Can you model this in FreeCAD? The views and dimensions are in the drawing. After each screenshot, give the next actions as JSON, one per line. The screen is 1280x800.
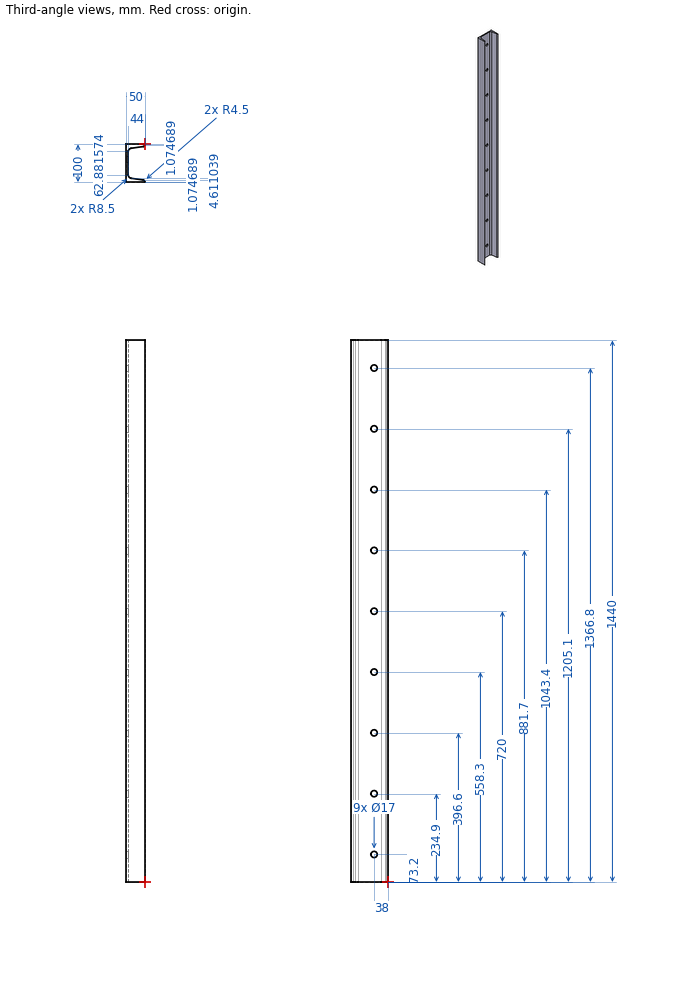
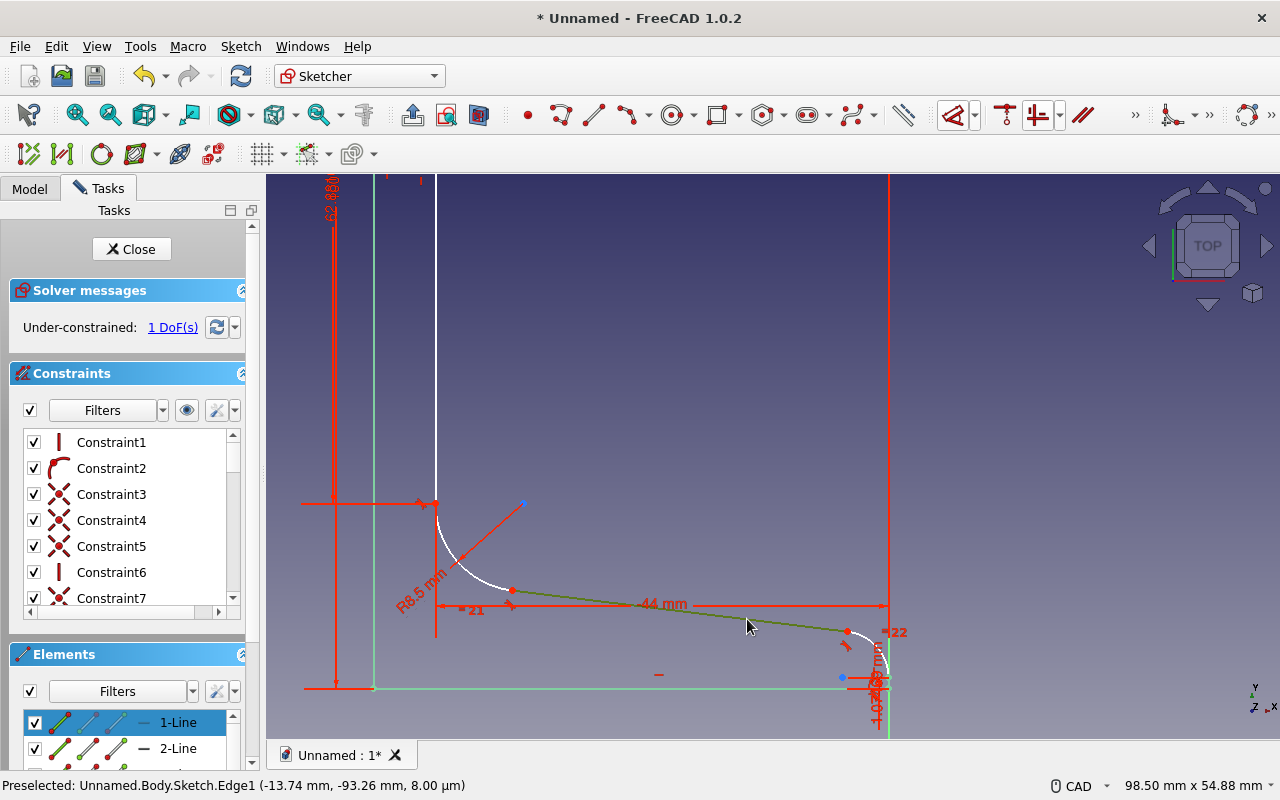
{"action": "left_click", "coordinate": [974, 116]}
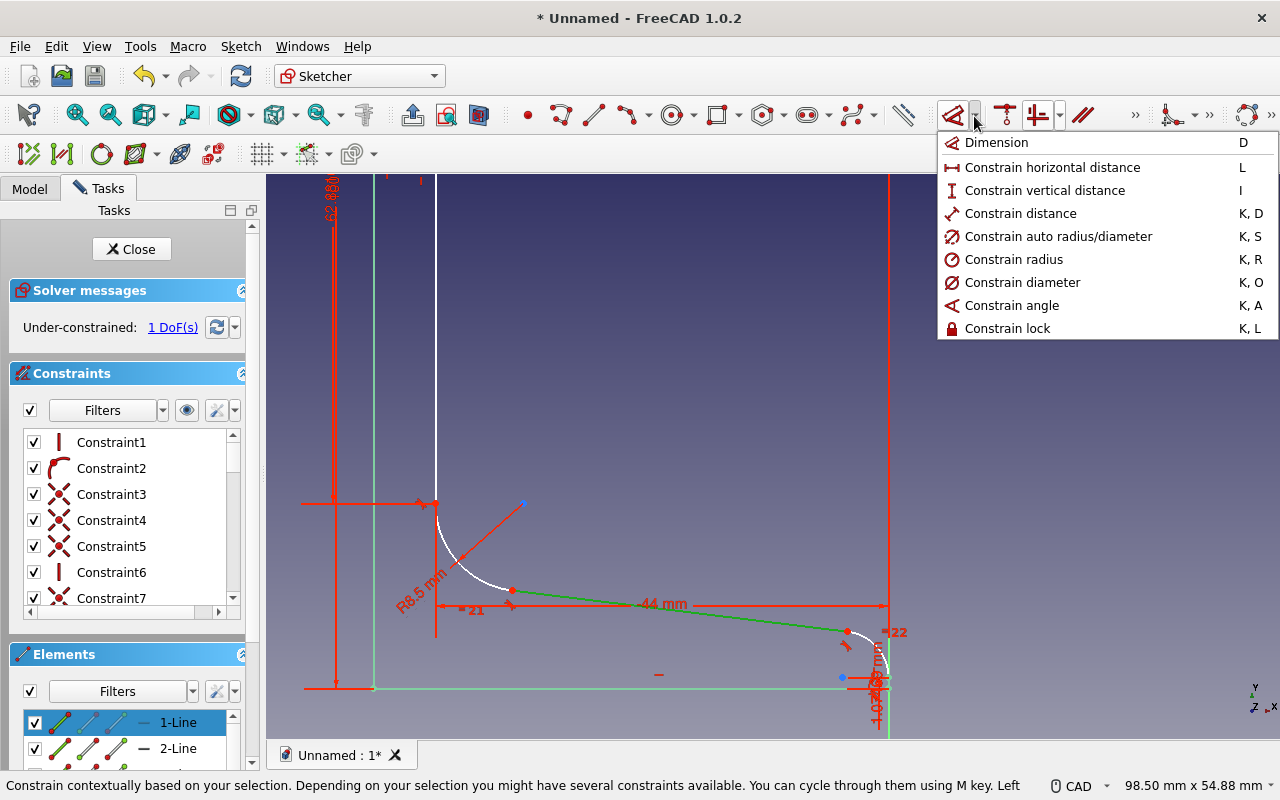
{"action": "left_click", "coordinate": [1108, 190]}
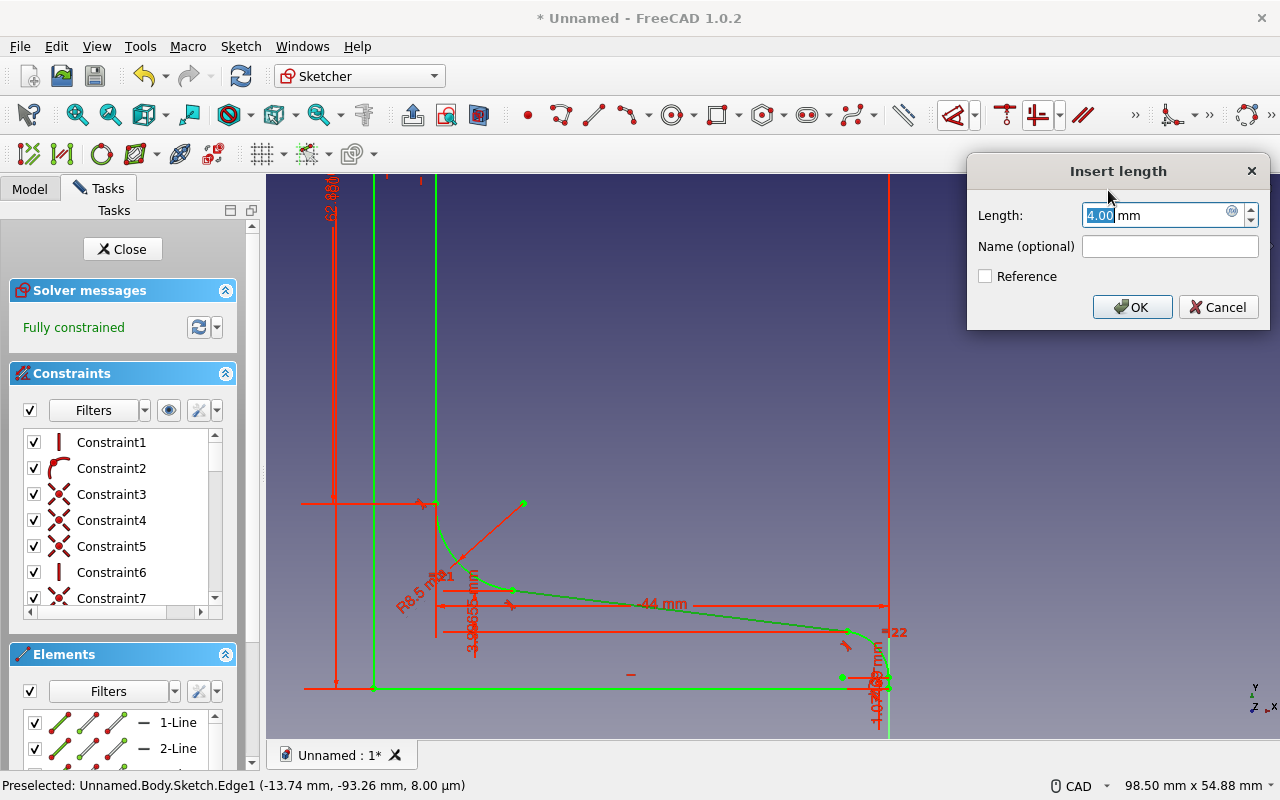
{"action": "type", "text": "4.611039"}
{"action": "key", "text": "Return"}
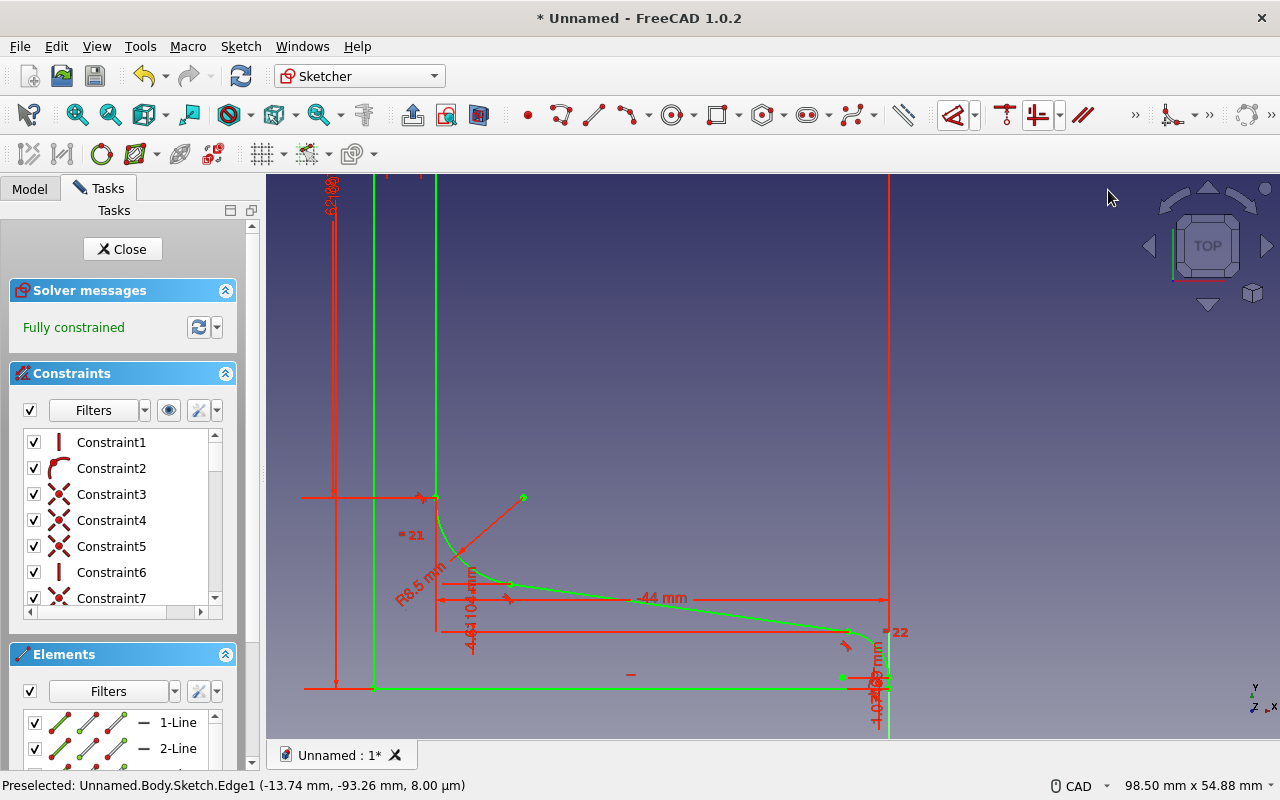
{"action": "left_click", "coordinate": [123, 249]}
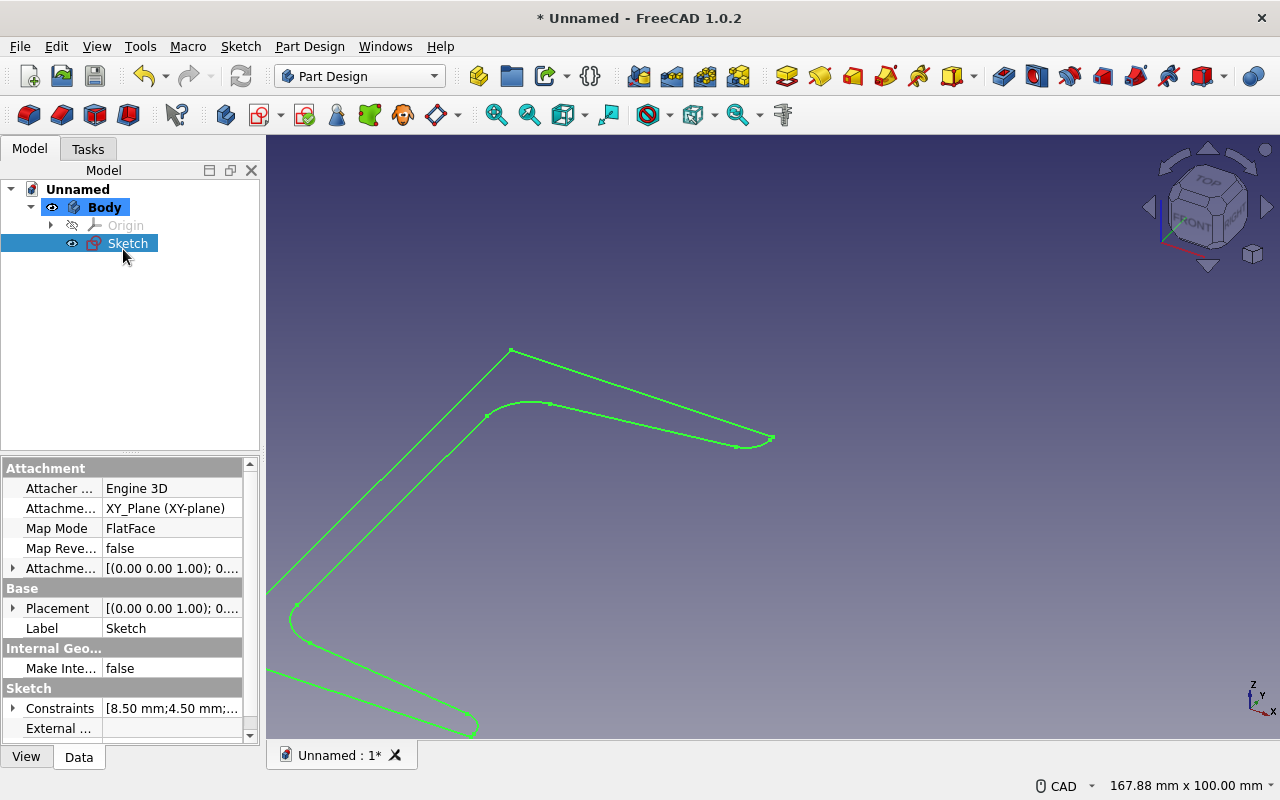
{"action": "left_click", "coordinate": [787, 76]}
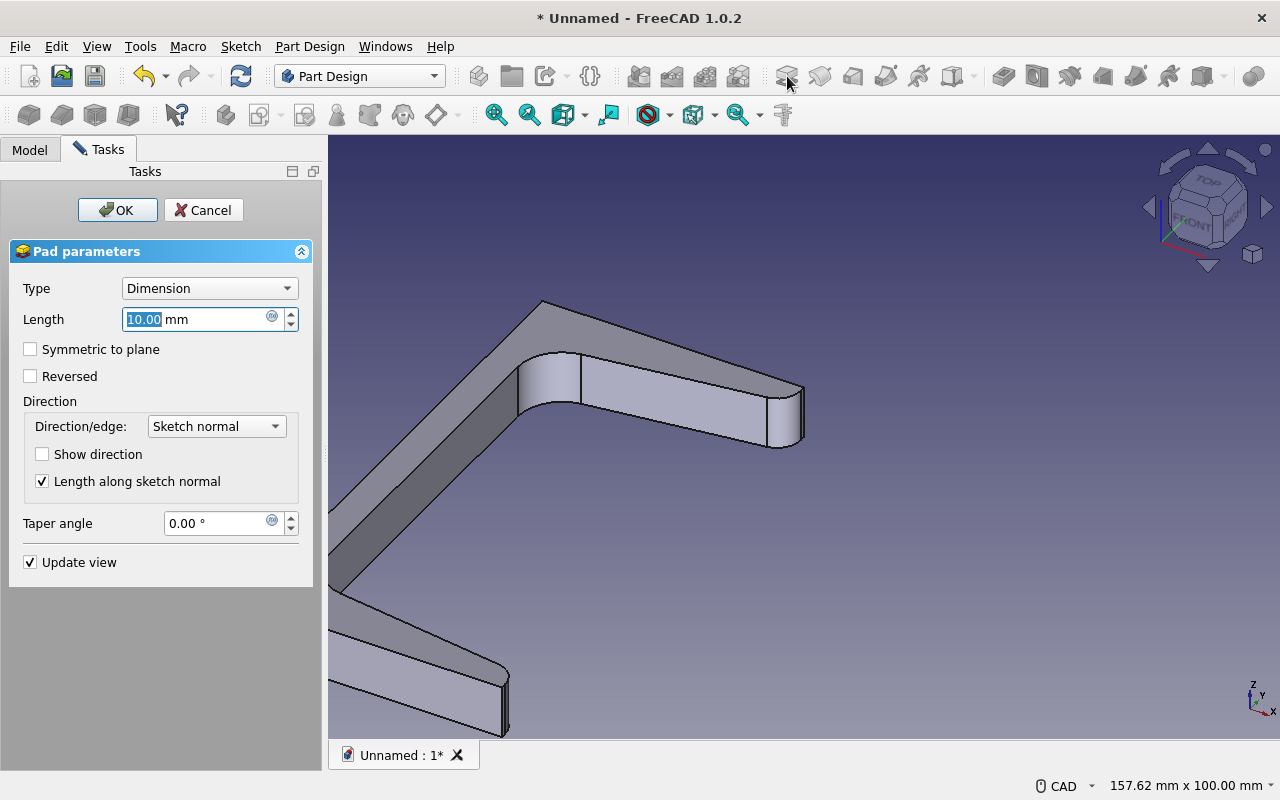
{"action": "type", "text": "1440"}
{"action": "key", "text": "Tab"}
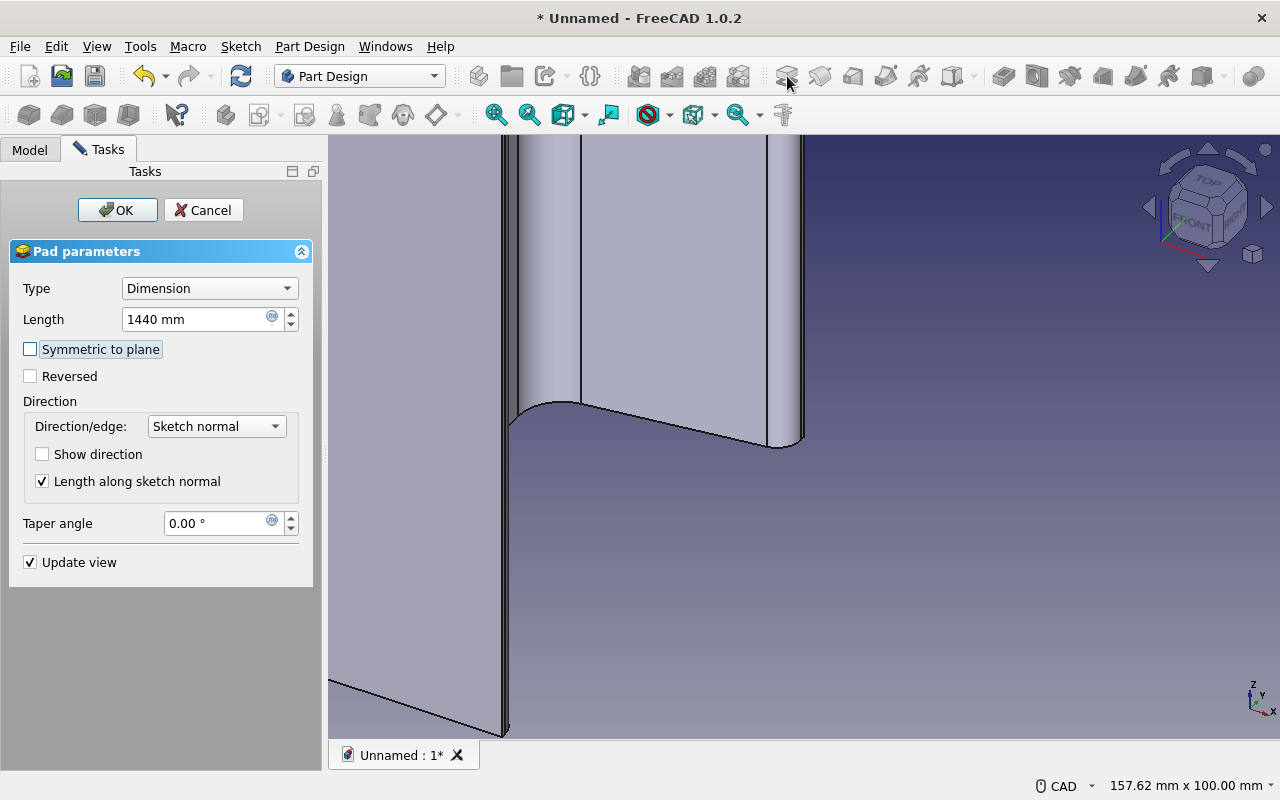
{"action": "left_click", "coordinate": [118, 210]}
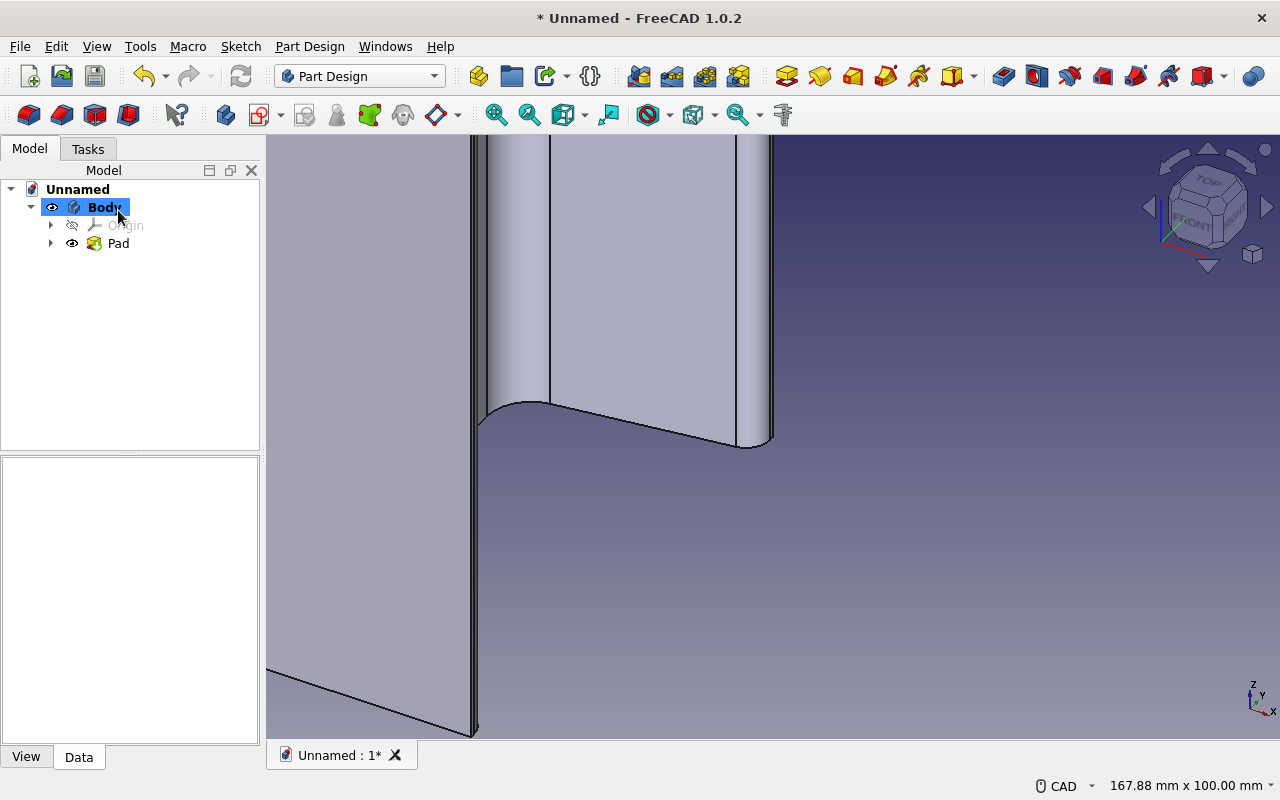
{"action": "left_click", "coordinate": [497, 116]}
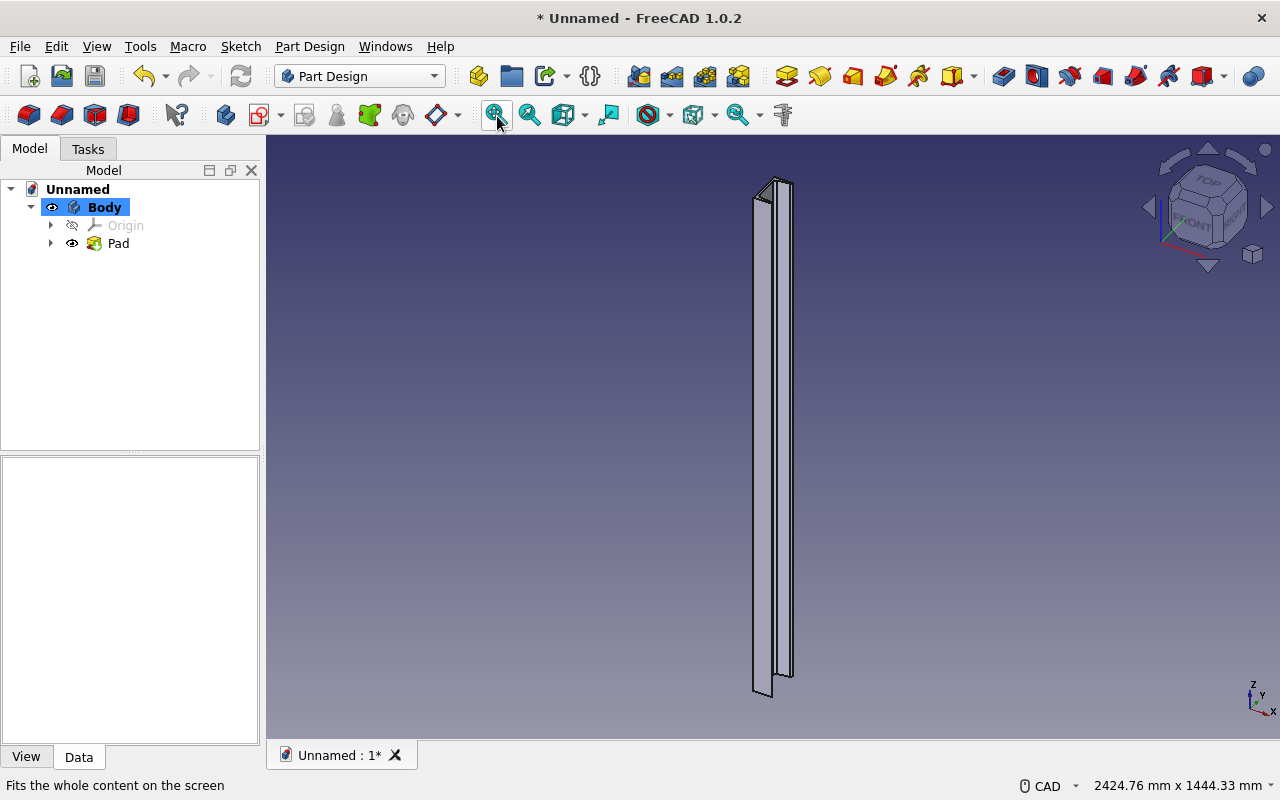
{"action": "key", "text": "6"}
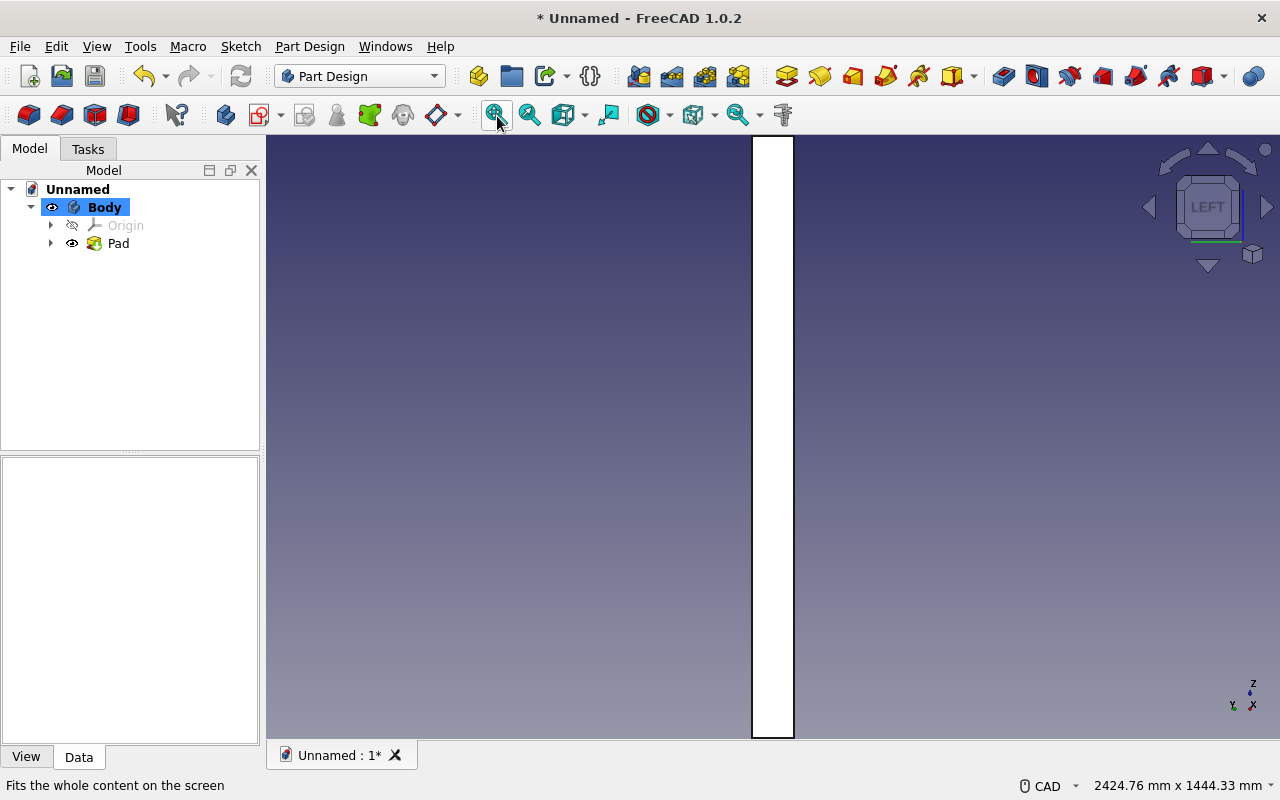
{"action": "left_click", "coordinate": [773, 178]}